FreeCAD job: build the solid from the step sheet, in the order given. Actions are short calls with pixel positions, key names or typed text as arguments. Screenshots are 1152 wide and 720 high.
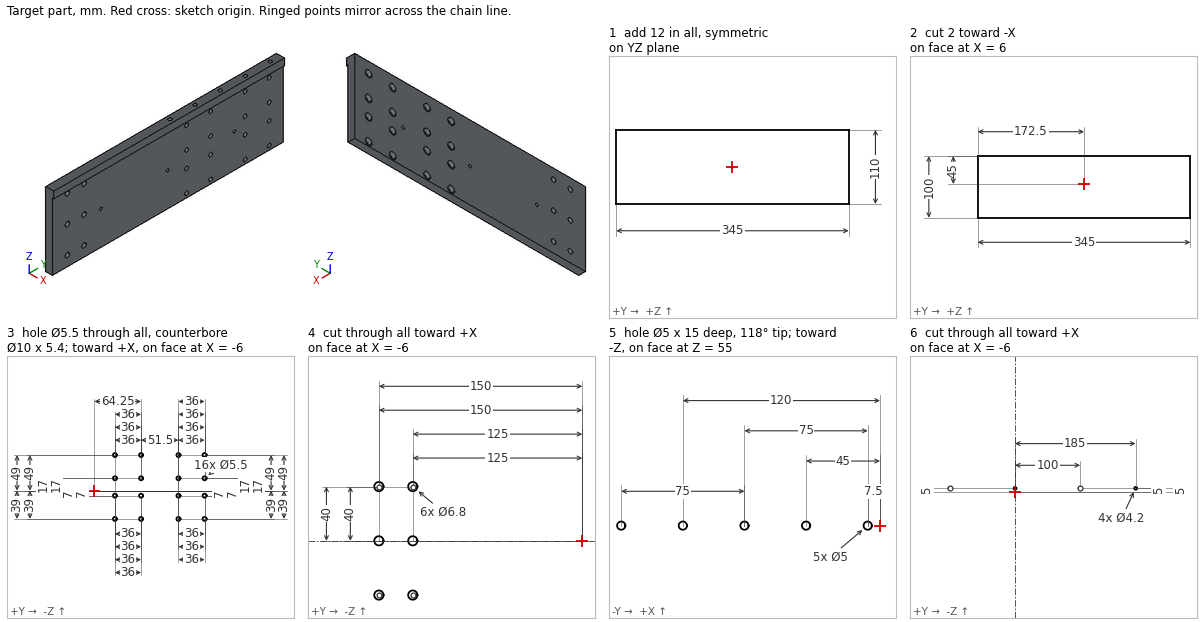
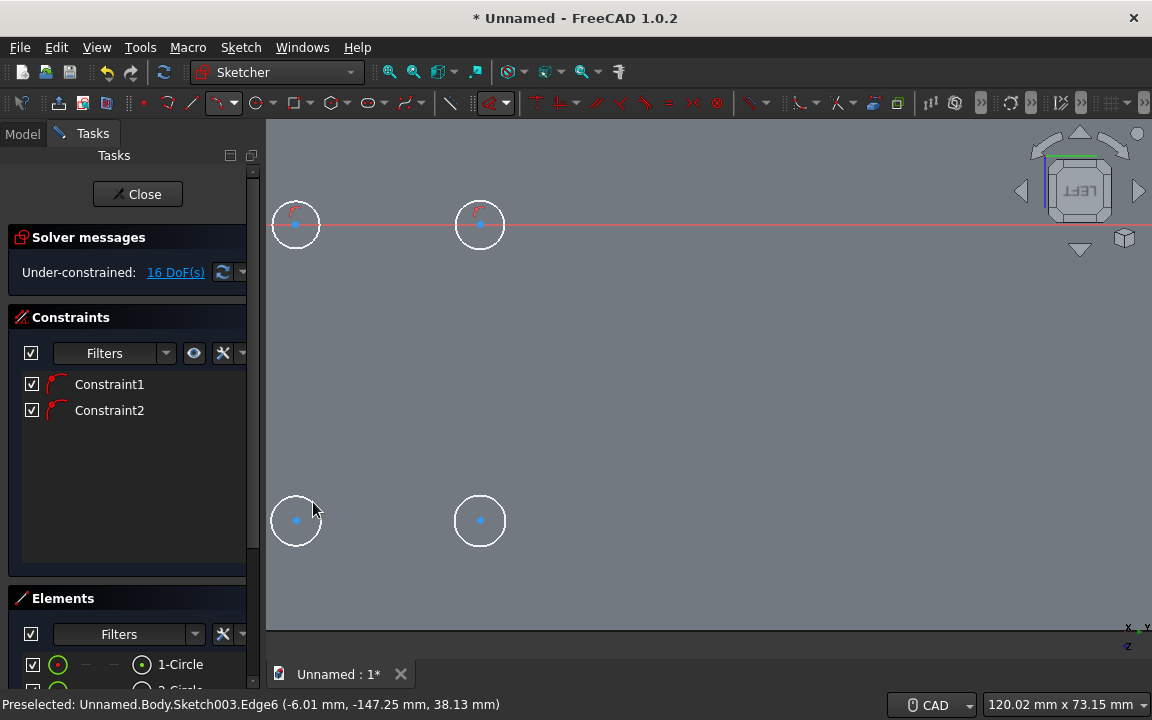
scroll(480, 523, down, 4)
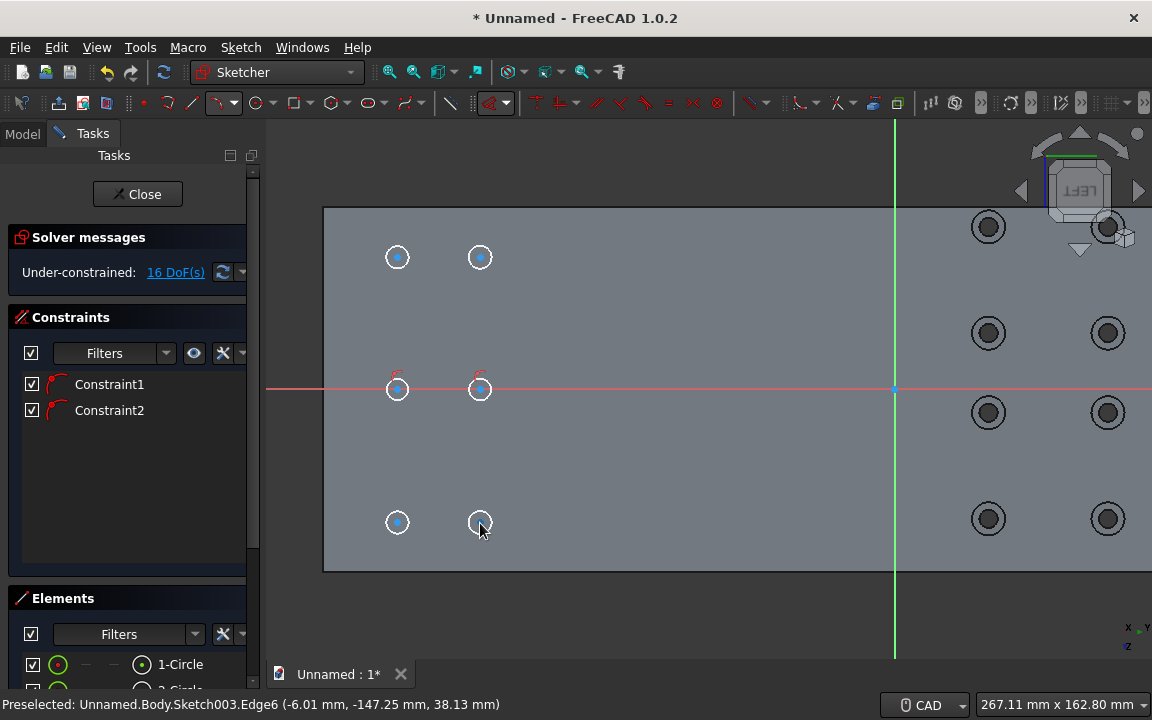
click(488, 249)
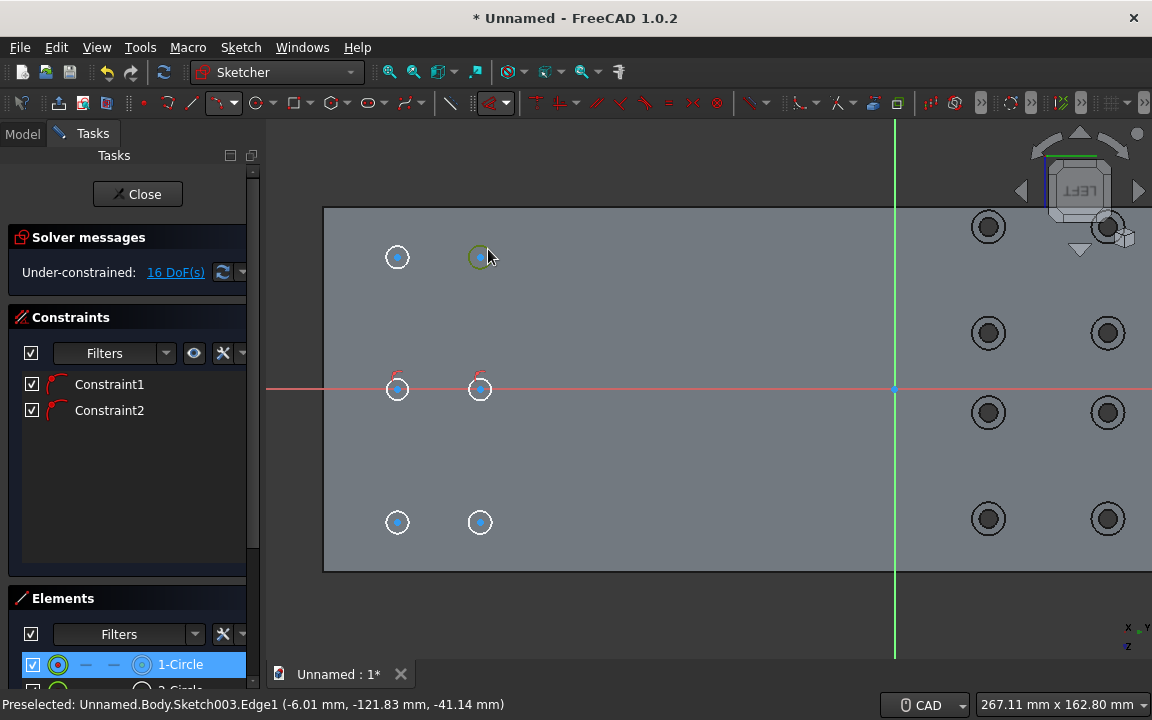
scroll(405, 249, up, 2)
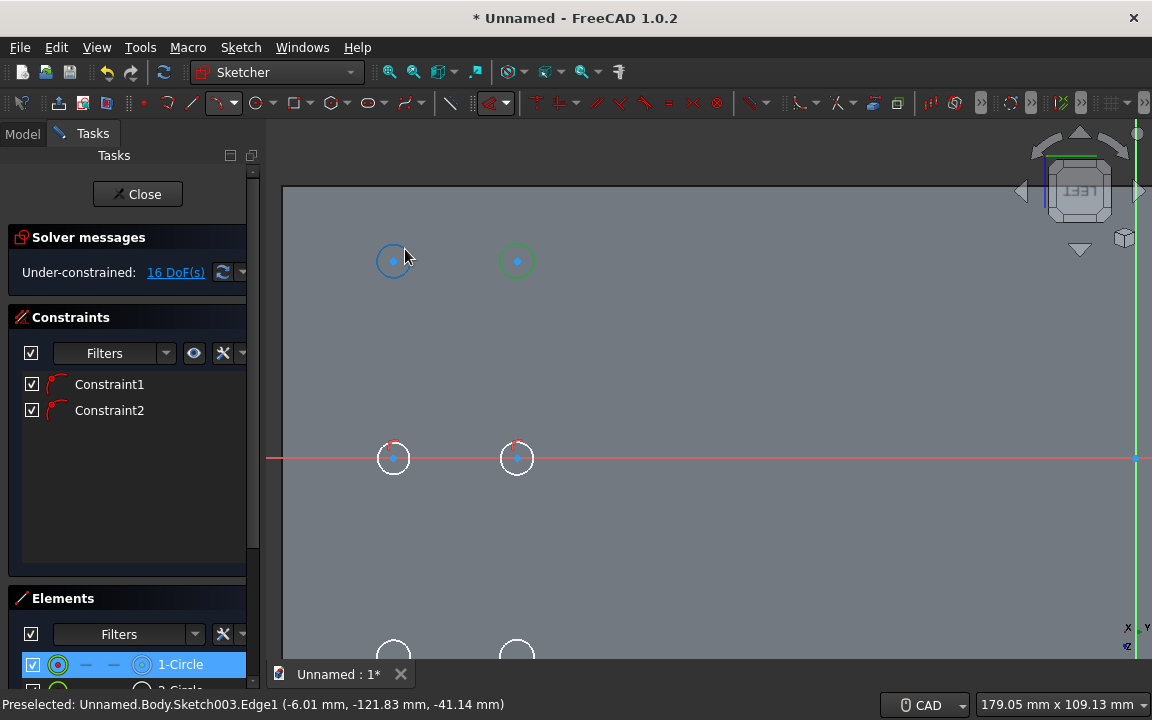
click(405, 249)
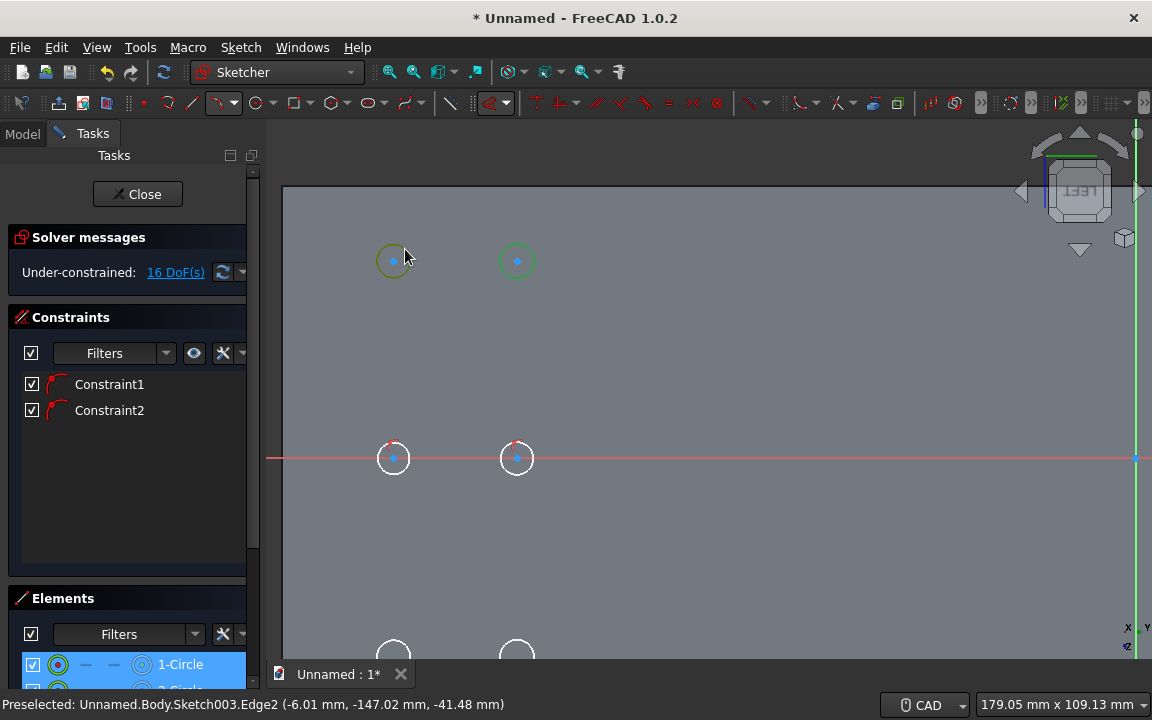
click(528, 447)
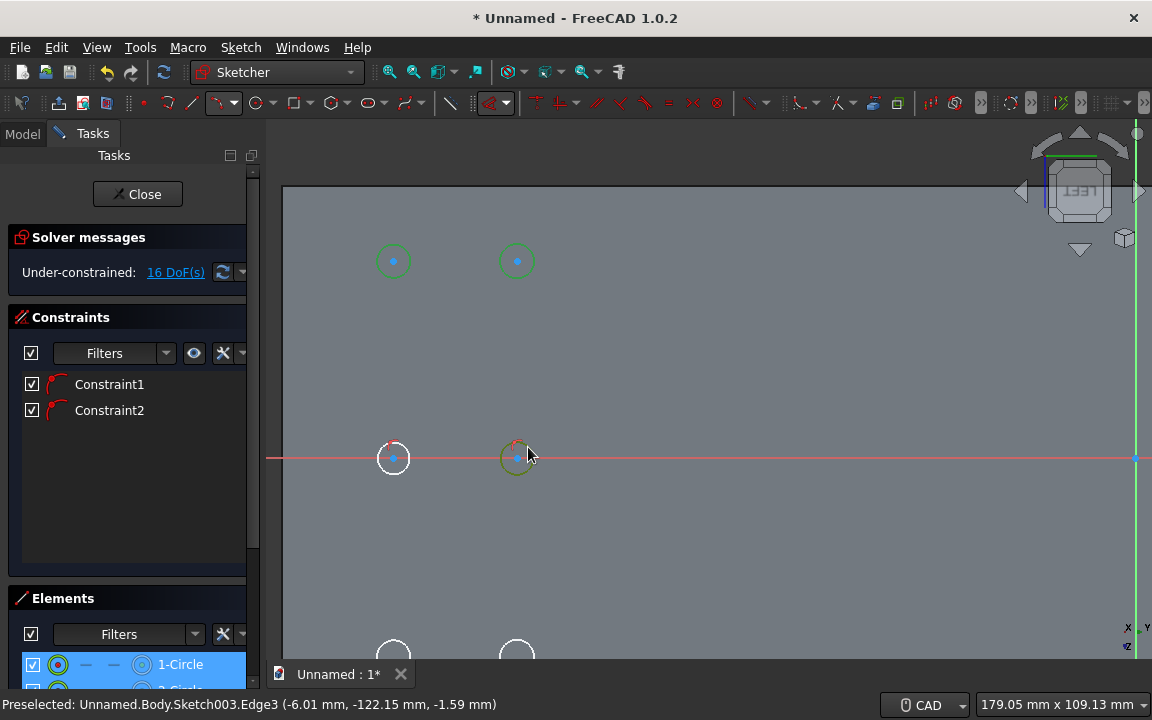
scroll(405, 447, up, 2)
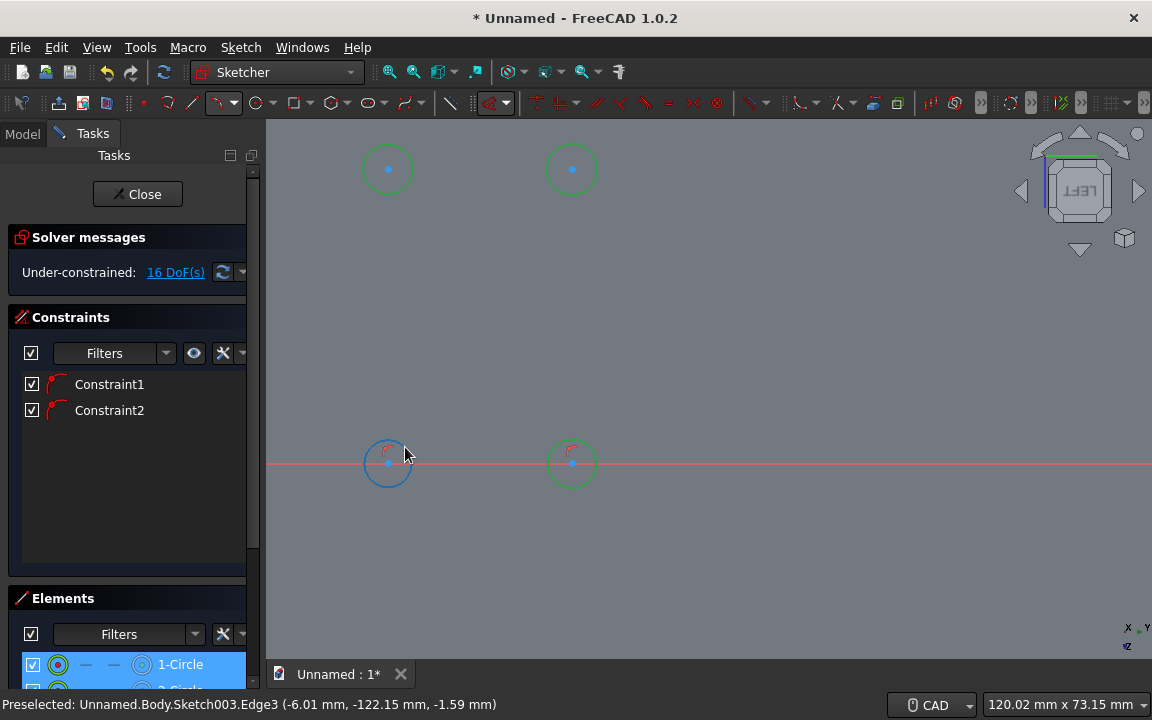
click(405, 447)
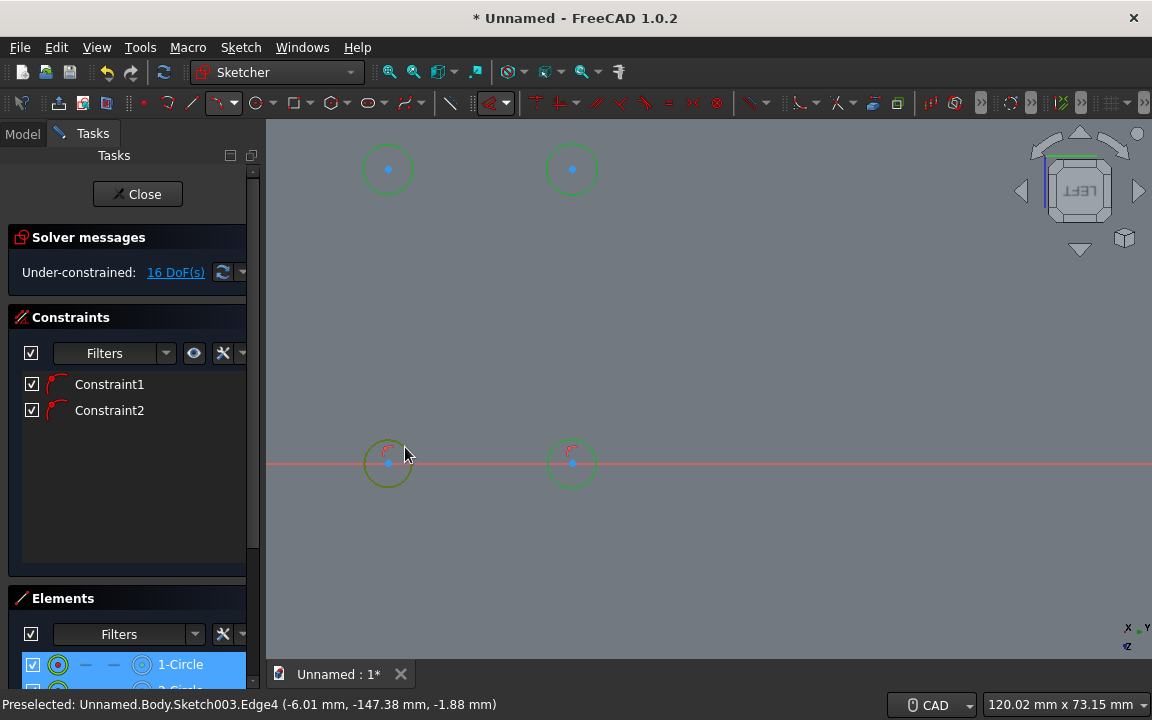
scroll(405, 328, down, 4)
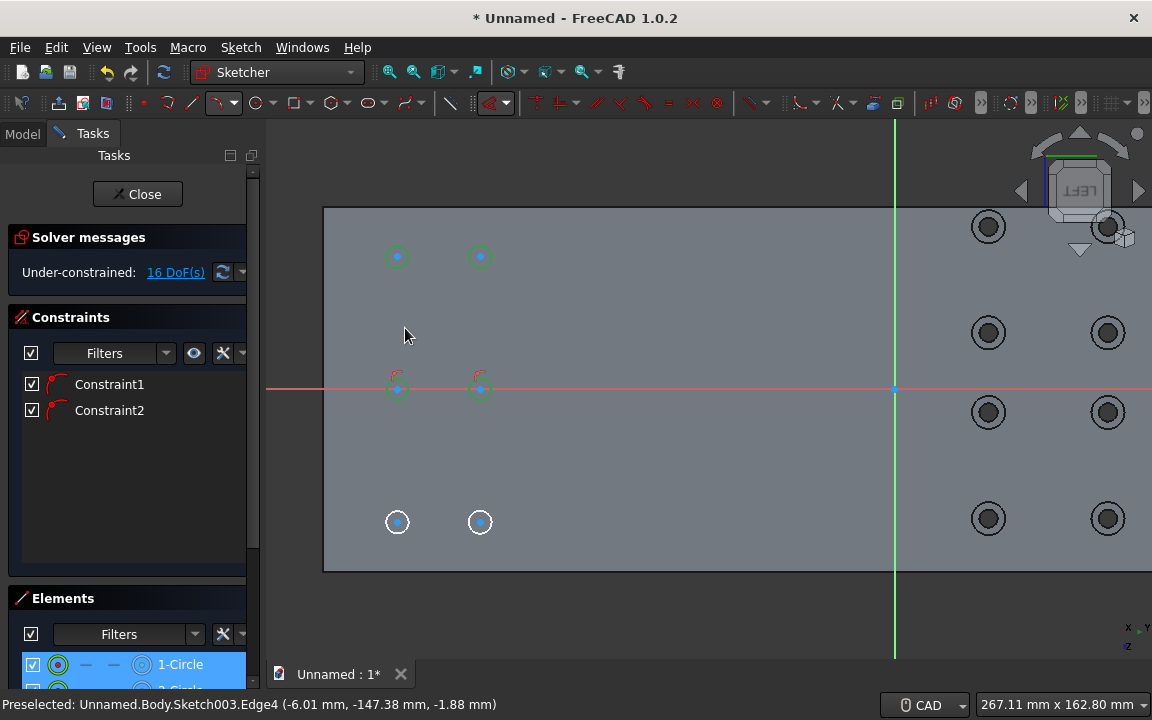
click(488, 514)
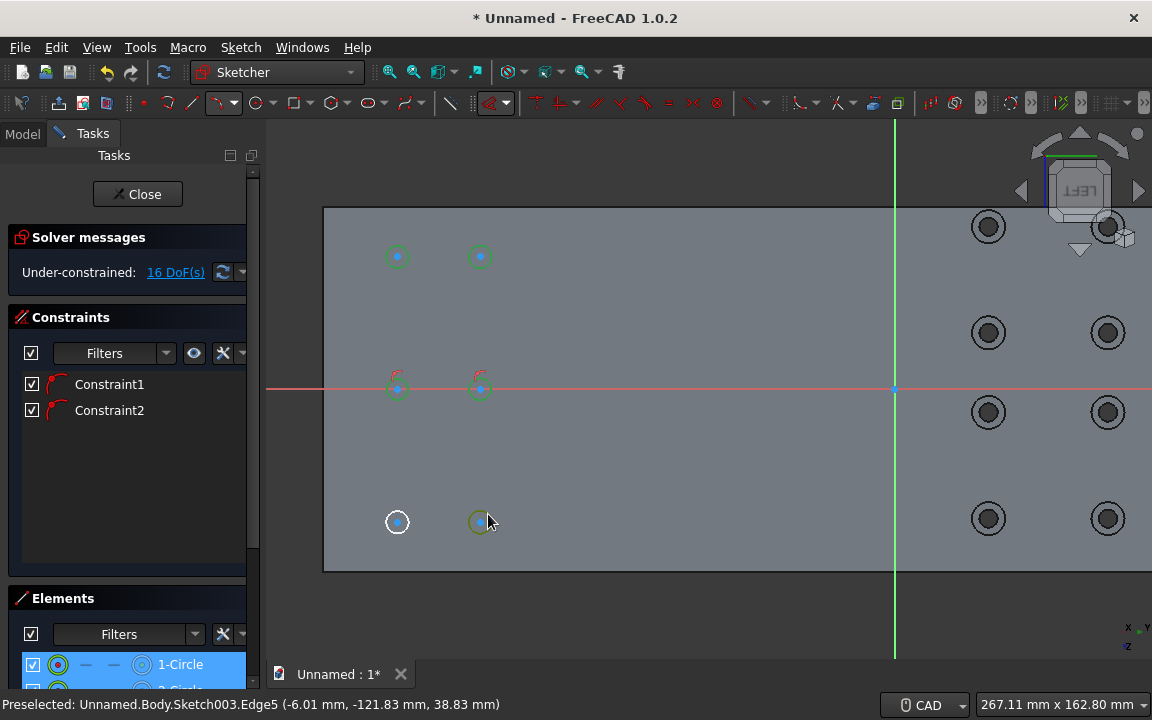
scroll(405, 514, up, 2)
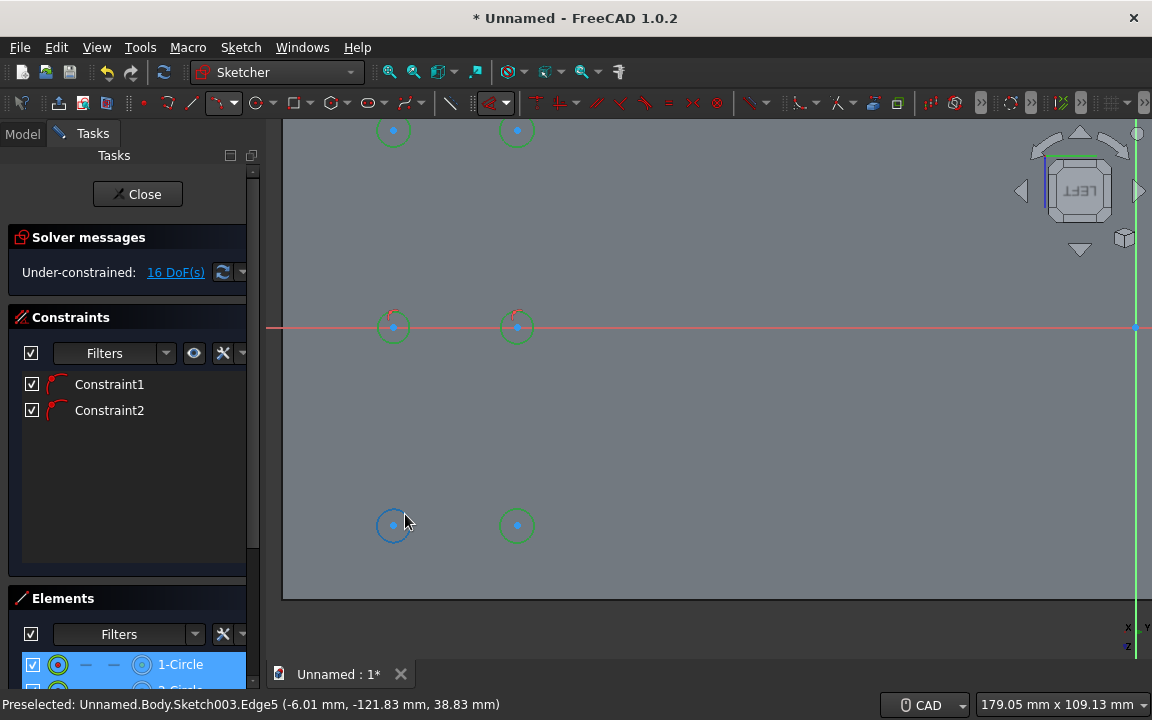
click(405, 514)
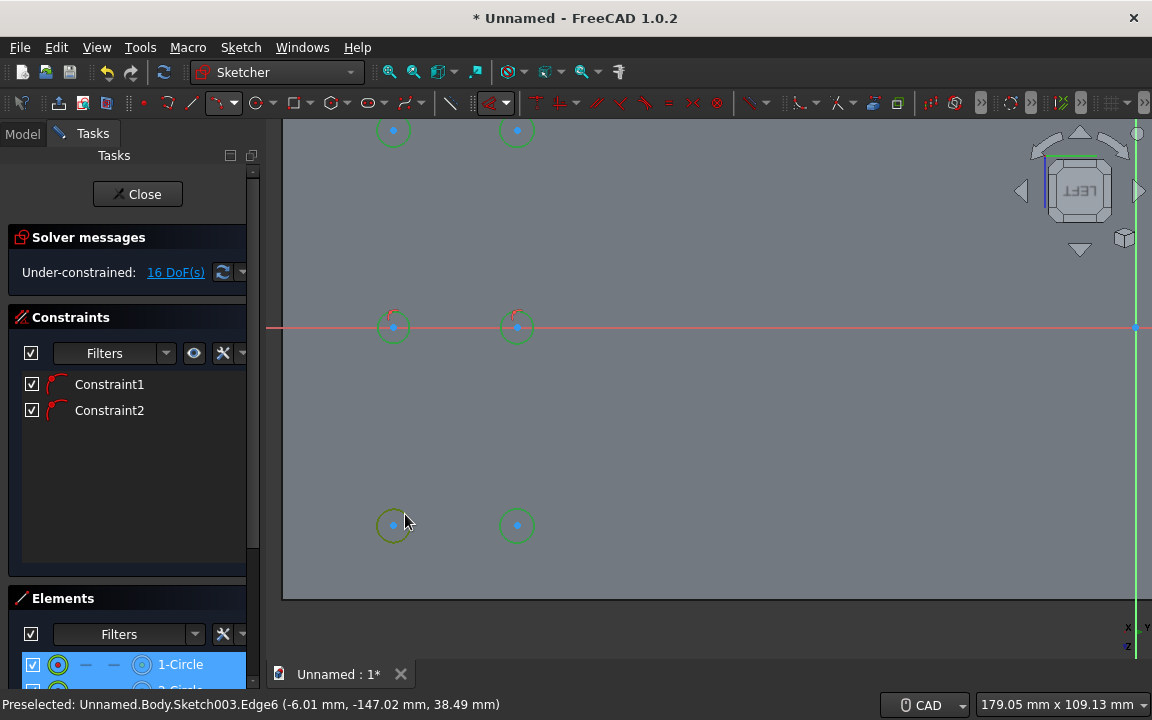
click(670, 104)